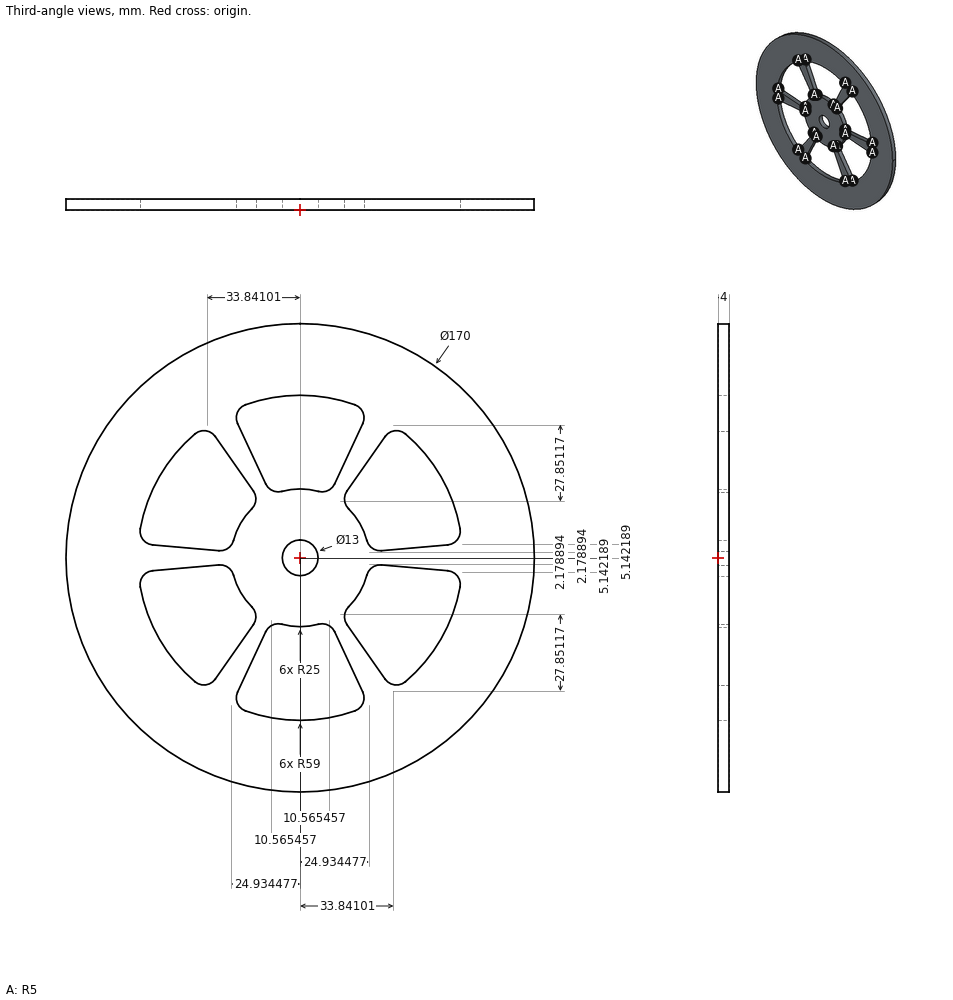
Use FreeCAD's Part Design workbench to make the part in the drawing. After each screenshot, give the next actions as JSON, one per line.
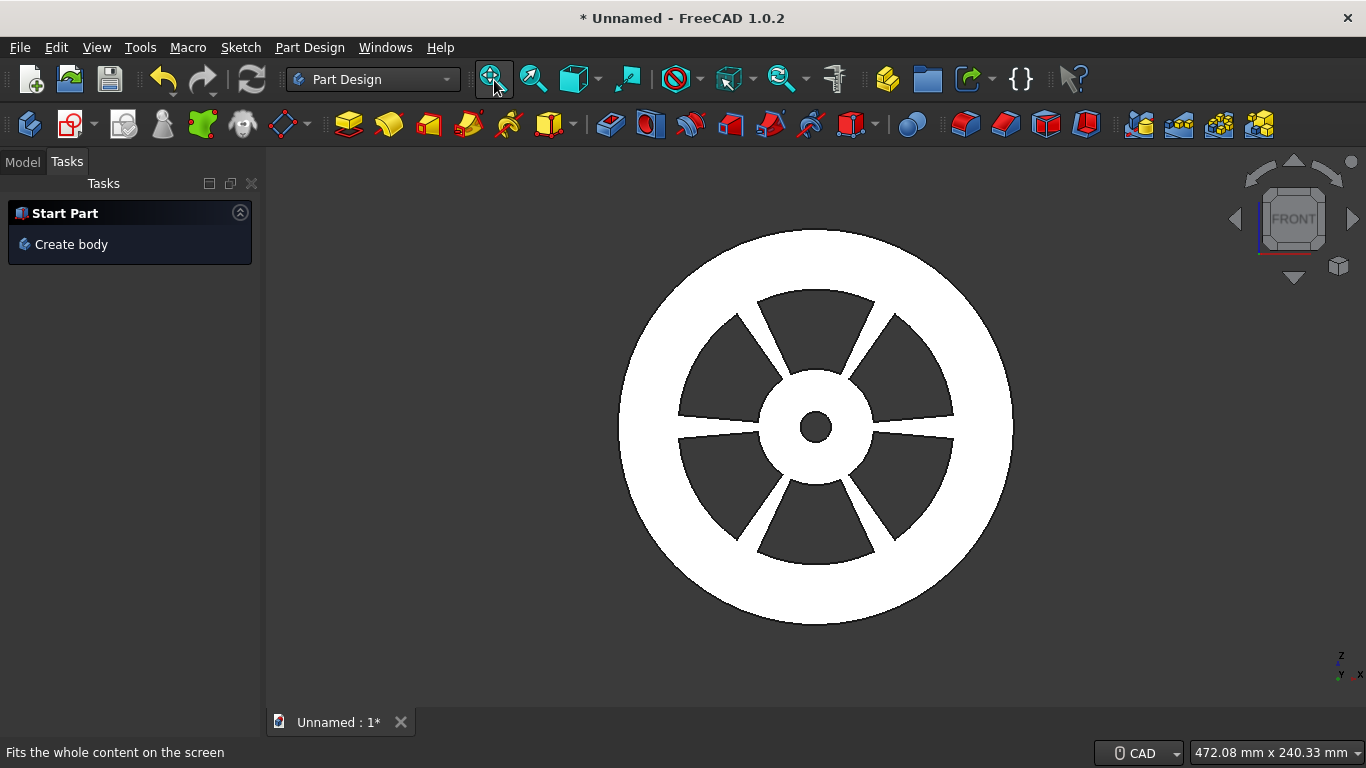
{"action": "scroll", "coordinate": [791, 373], "scroll_direction": "up", "scroll_amount": 8}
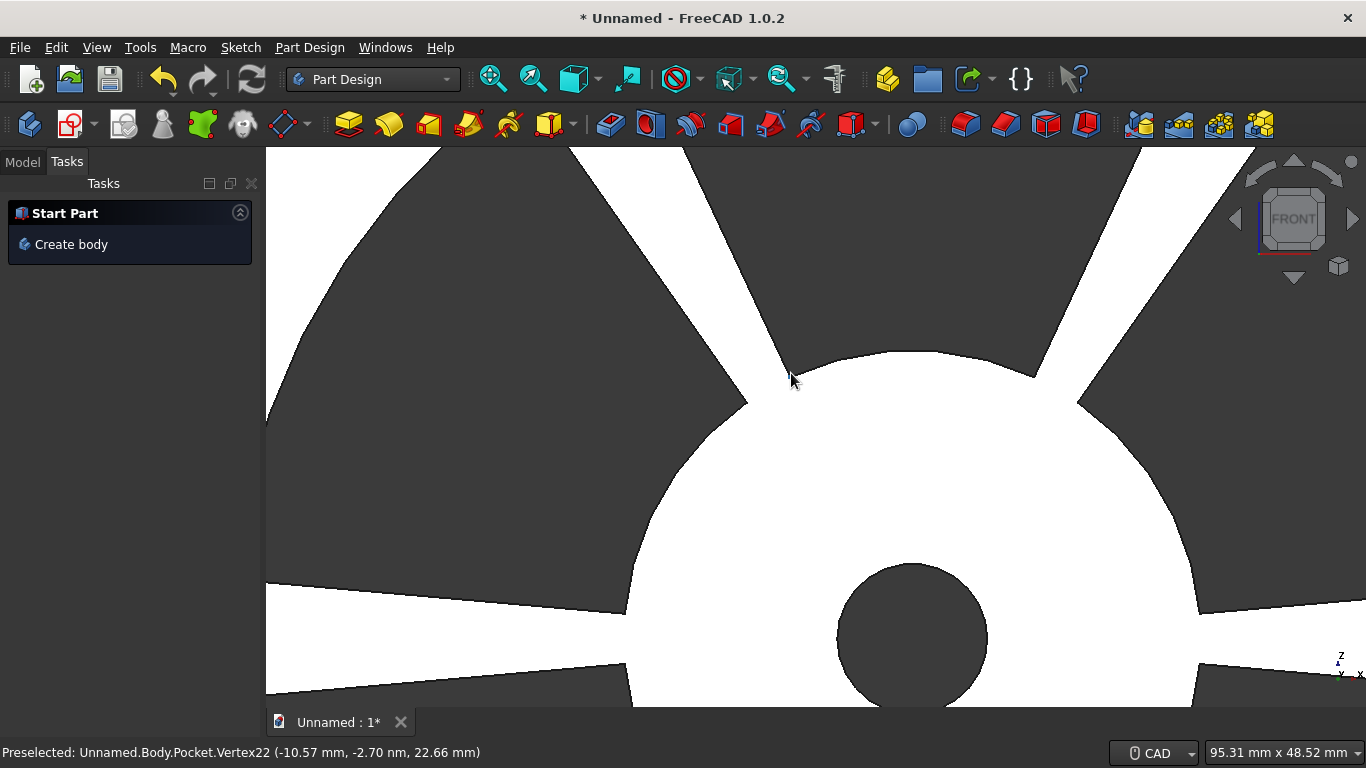
{"action": "left_click", "coordinate": [494, 80]}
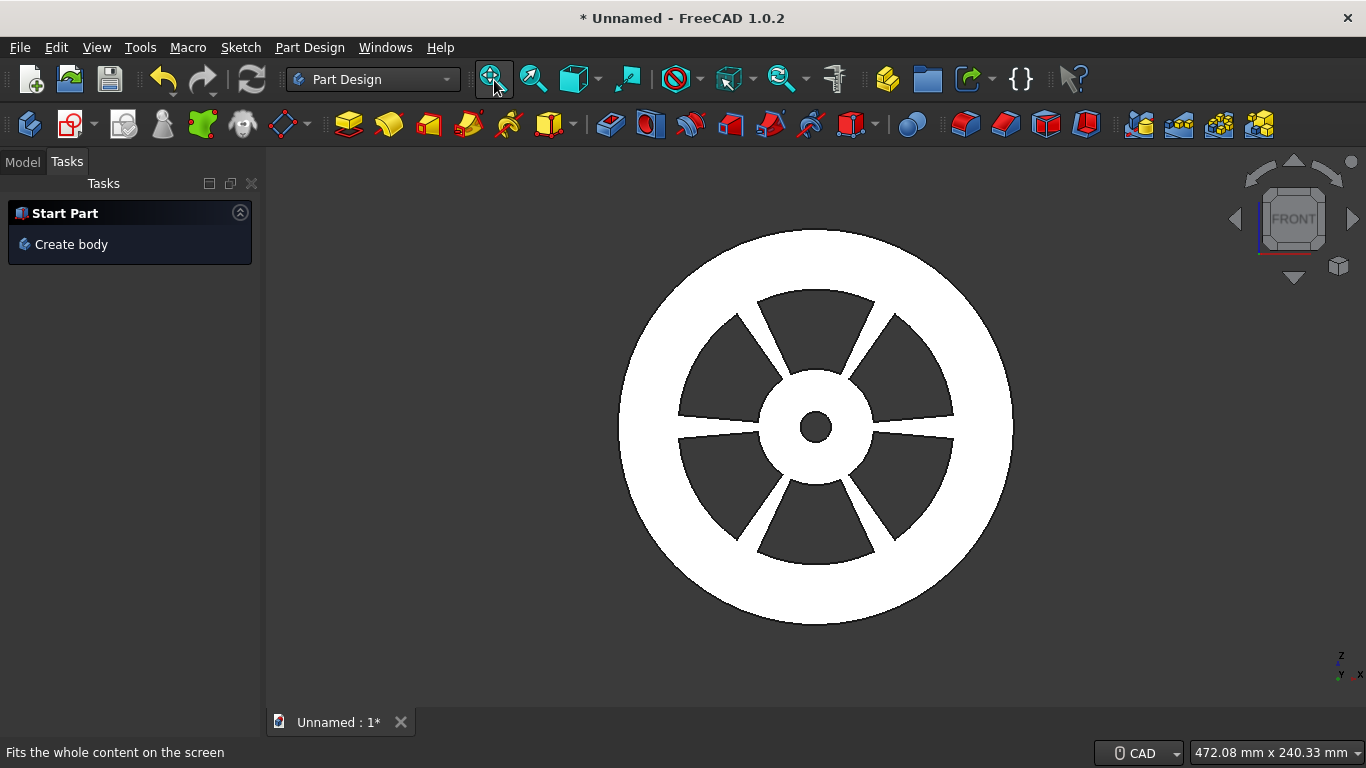
{"action": "key", "text": "3"}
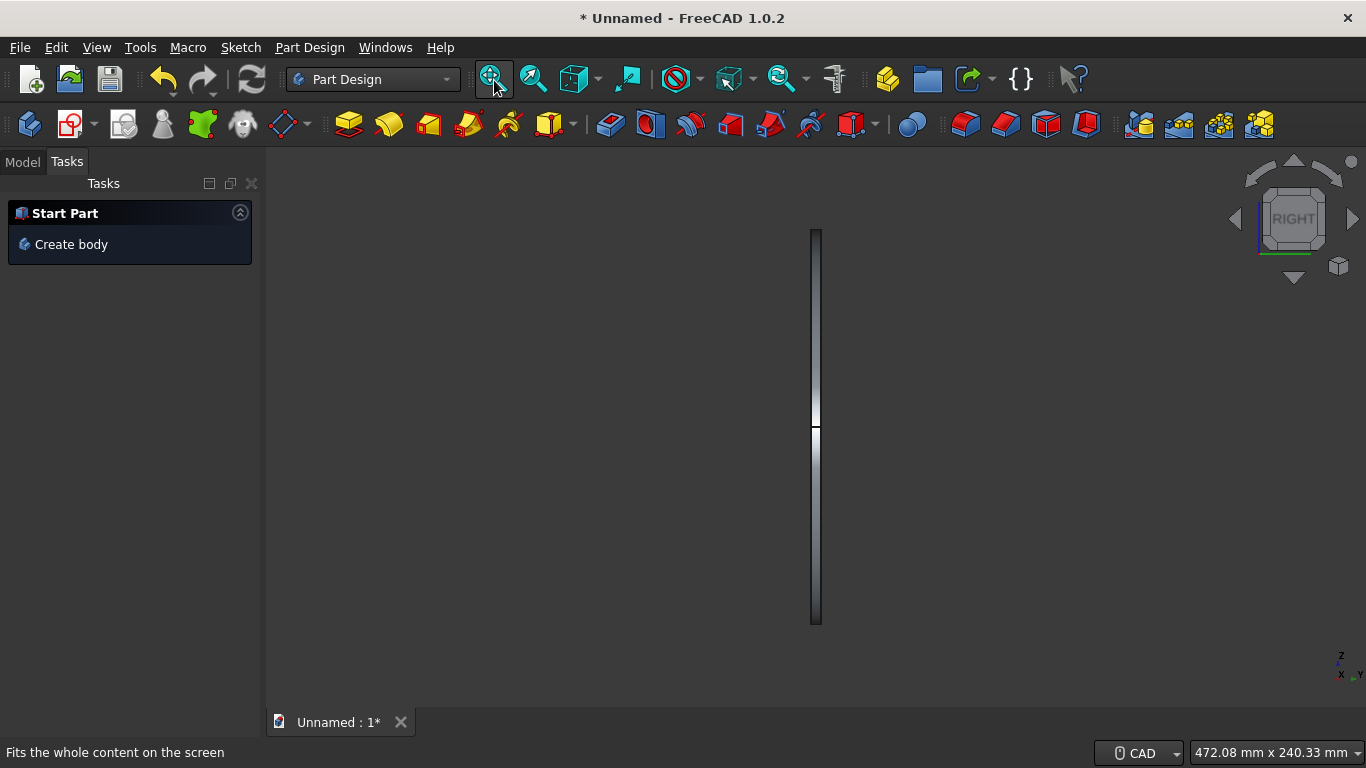
{"action": "scroll", "coordinate": [816, 373], "scroll_direction": "up", "scroll_amount": 8}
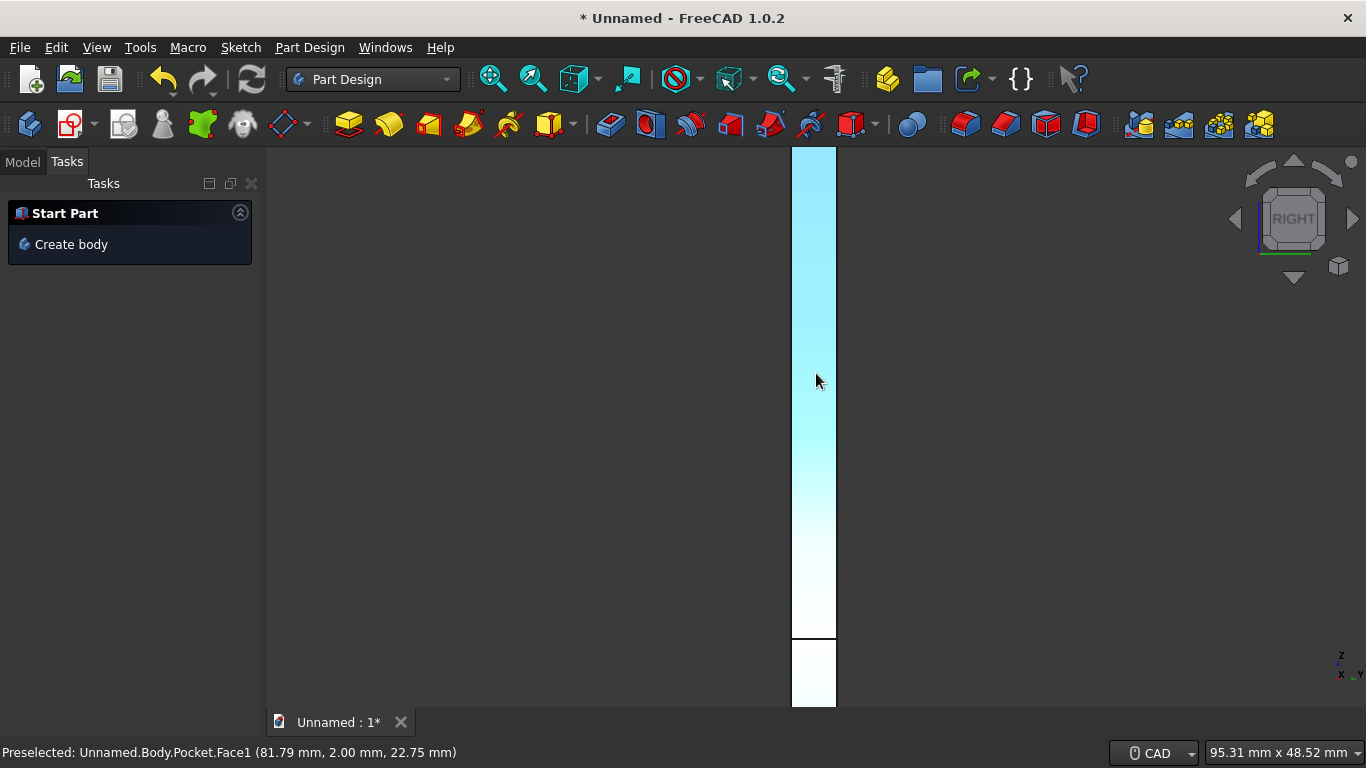
{"action": "left_click", "coordinate": [494, 80]}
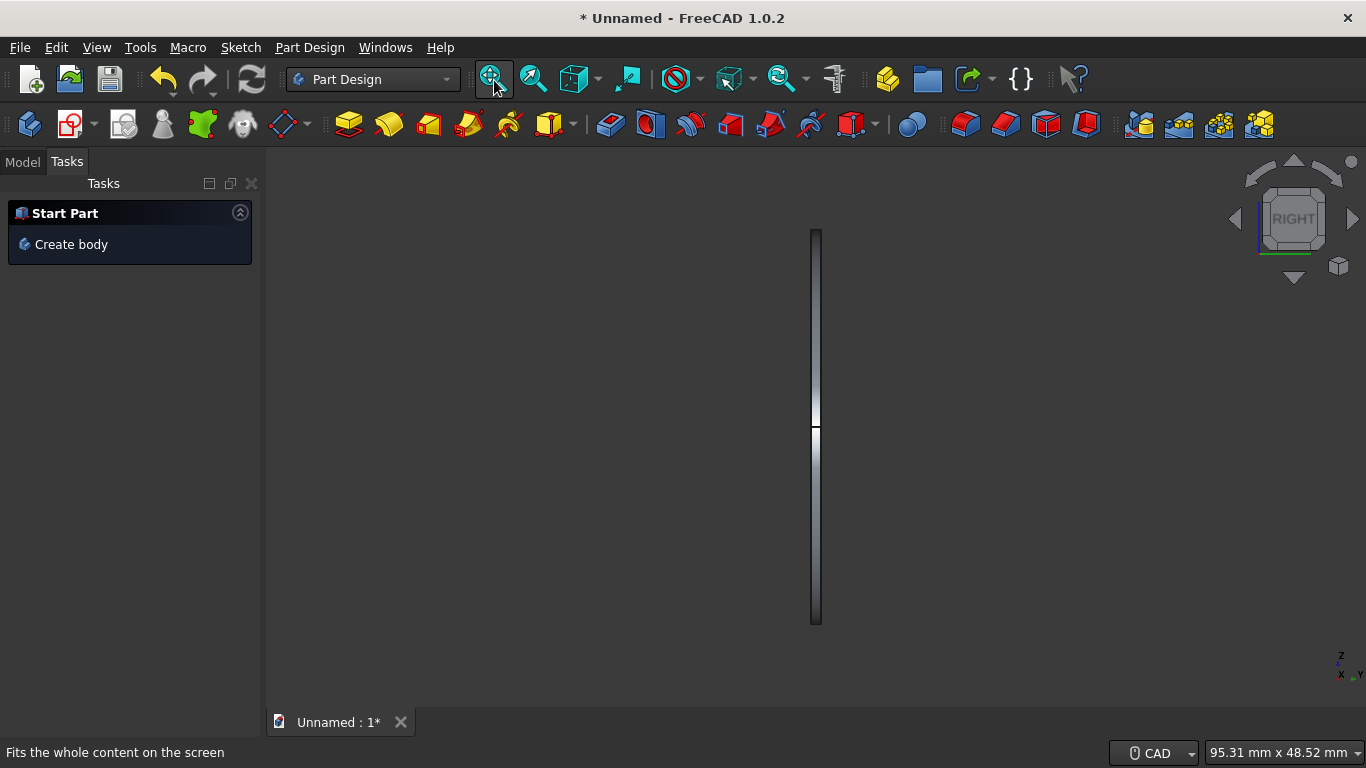
{"action": "key", "text": "5"}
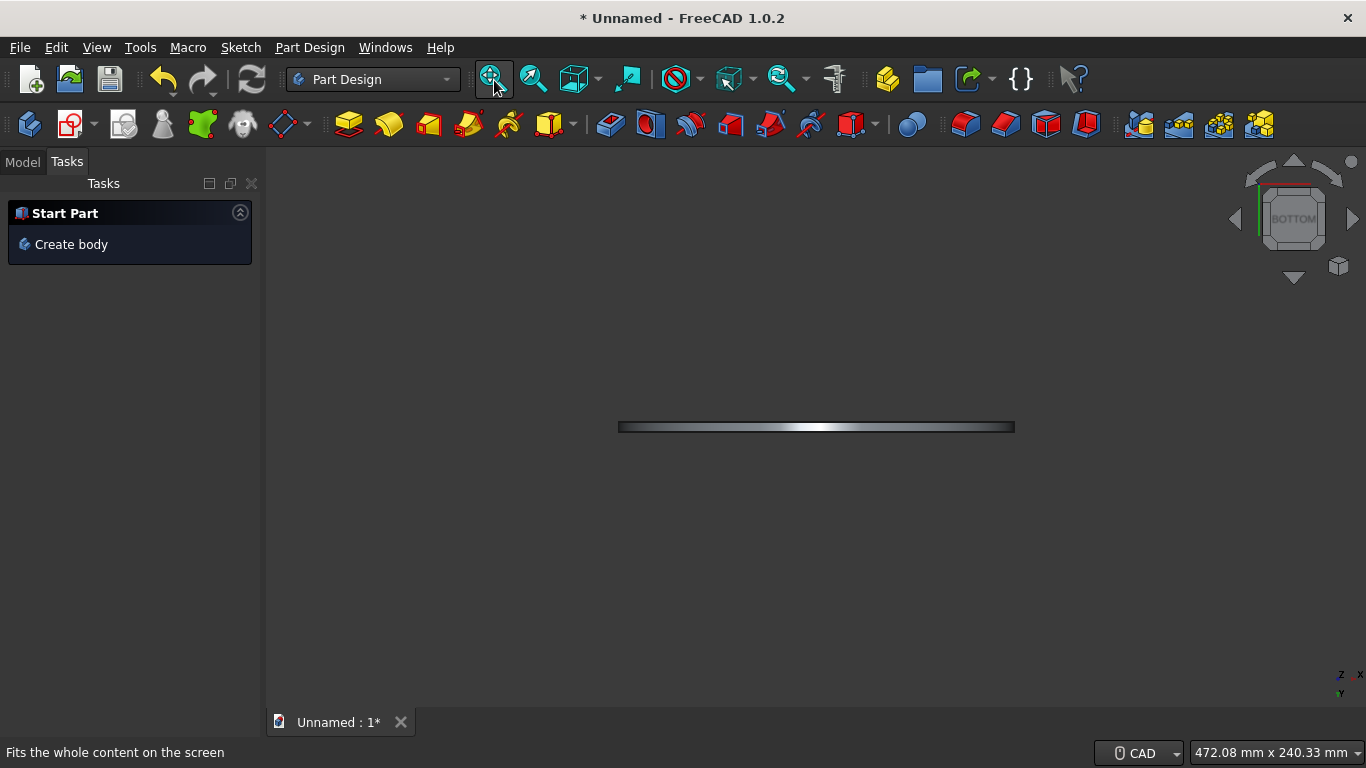
{"action": "left_click", "coordinate": [494, 80]}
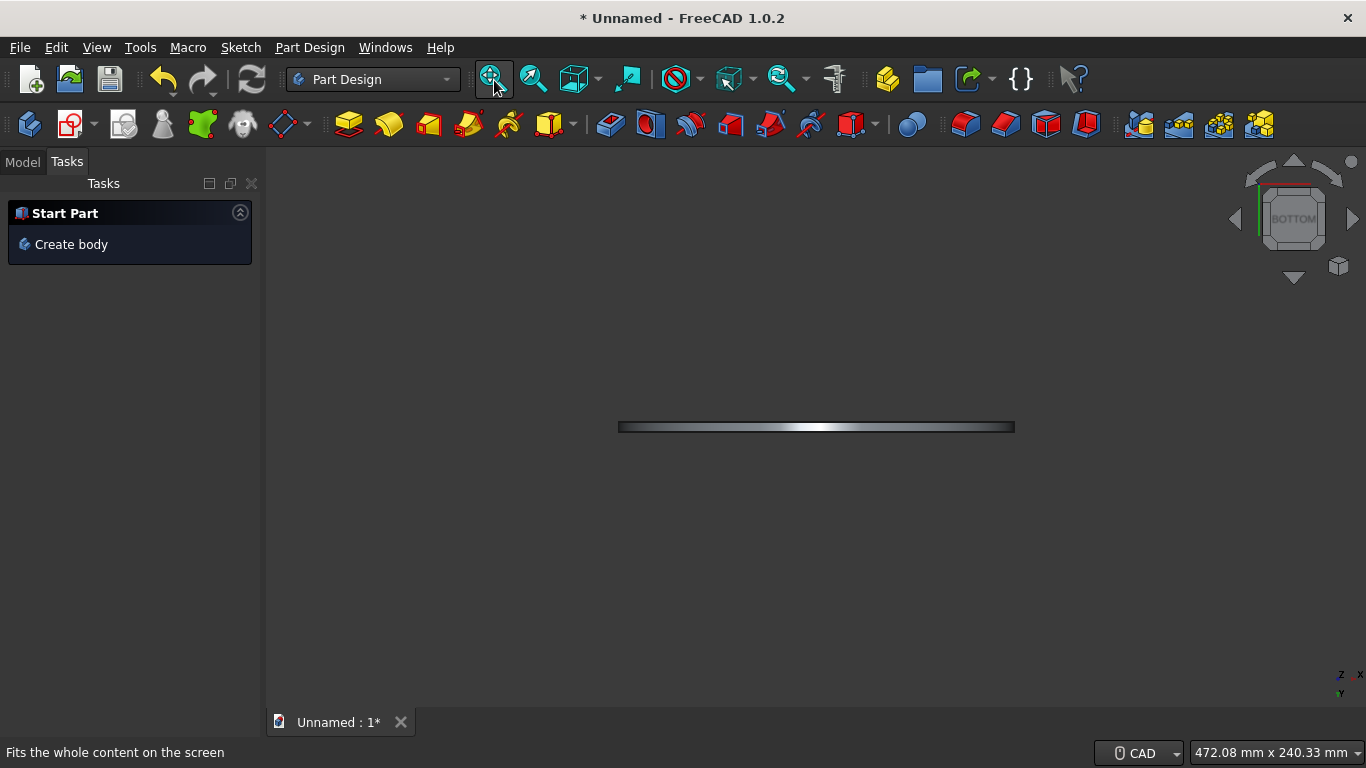
{"action": "scroll", "coordinate": [791, 426], "scroll_direction": "up", "scroll_amount": 8}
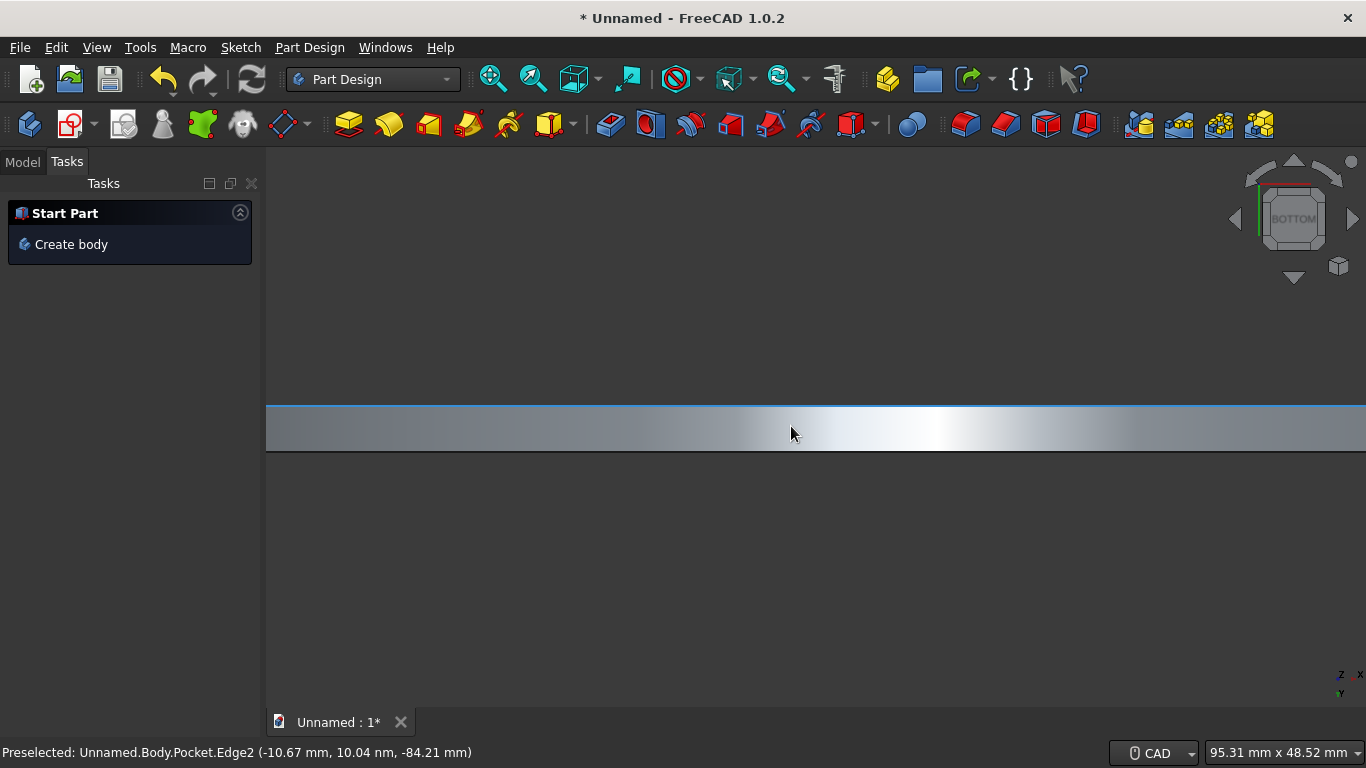
{"action": "left_click", "coordinate": [494, 80]}